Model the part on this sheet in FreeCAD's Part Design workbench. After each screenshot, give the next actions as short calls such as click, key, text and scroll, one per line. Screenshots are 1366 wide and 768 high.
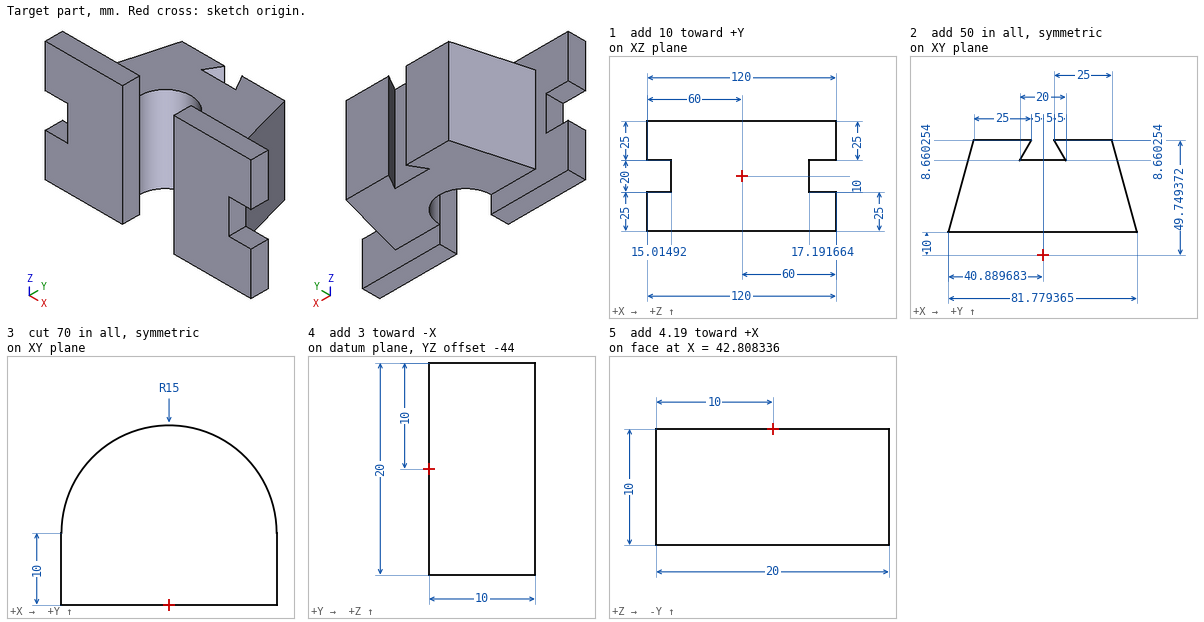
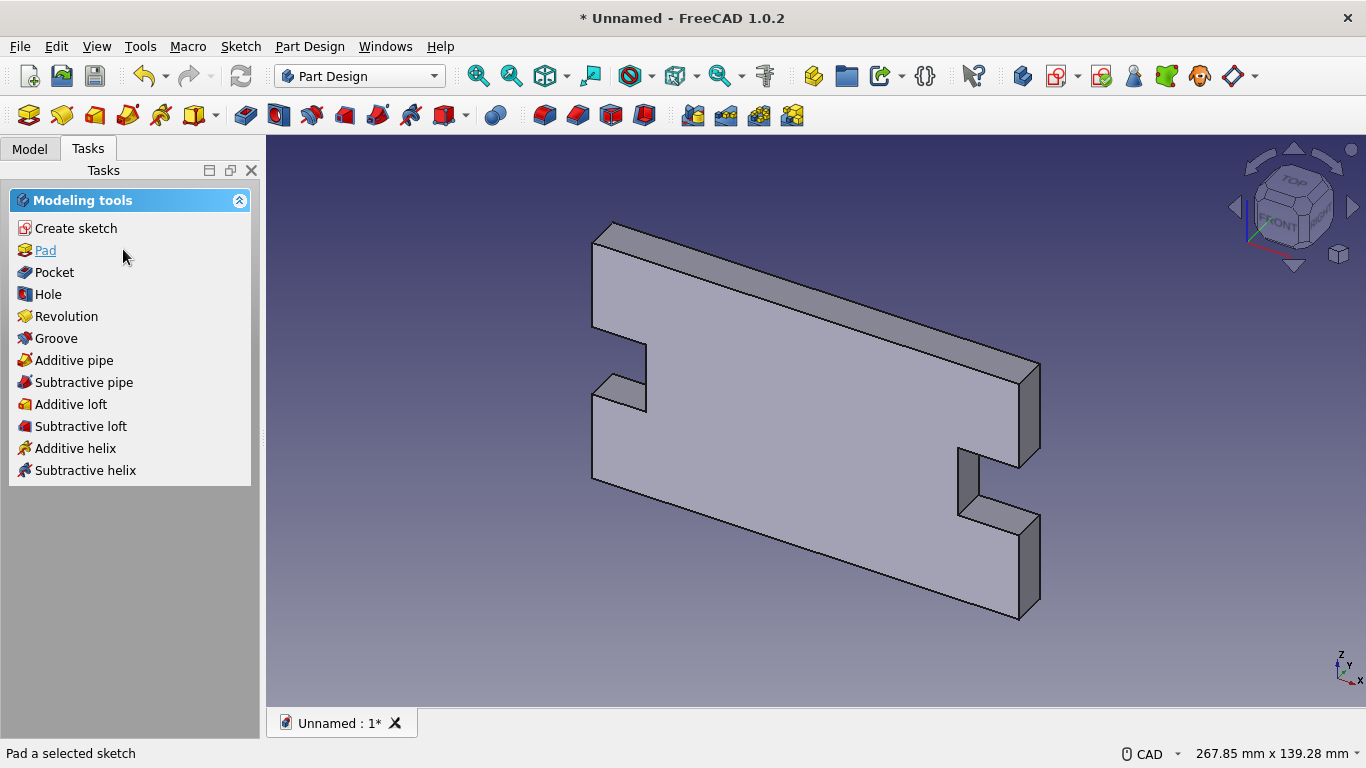
click(29, 116)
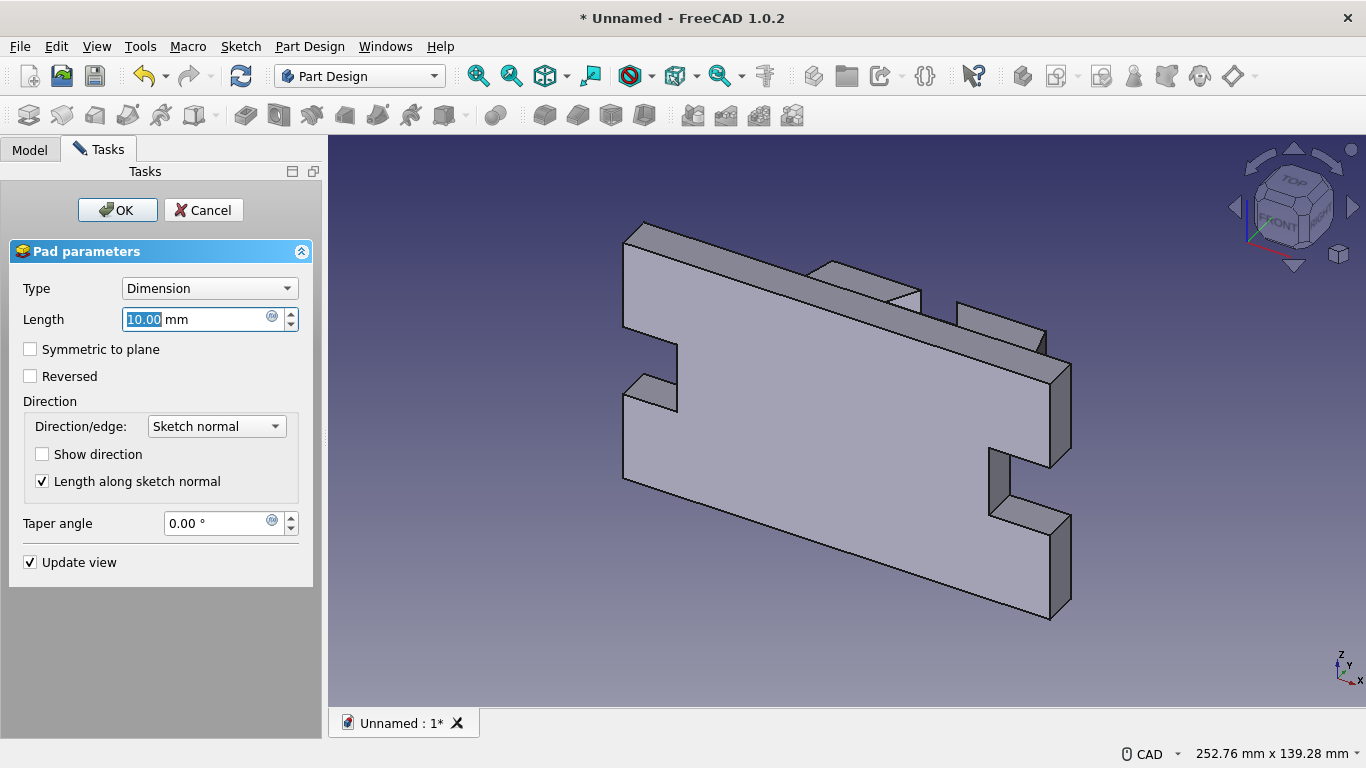
text(50)
key(Tab)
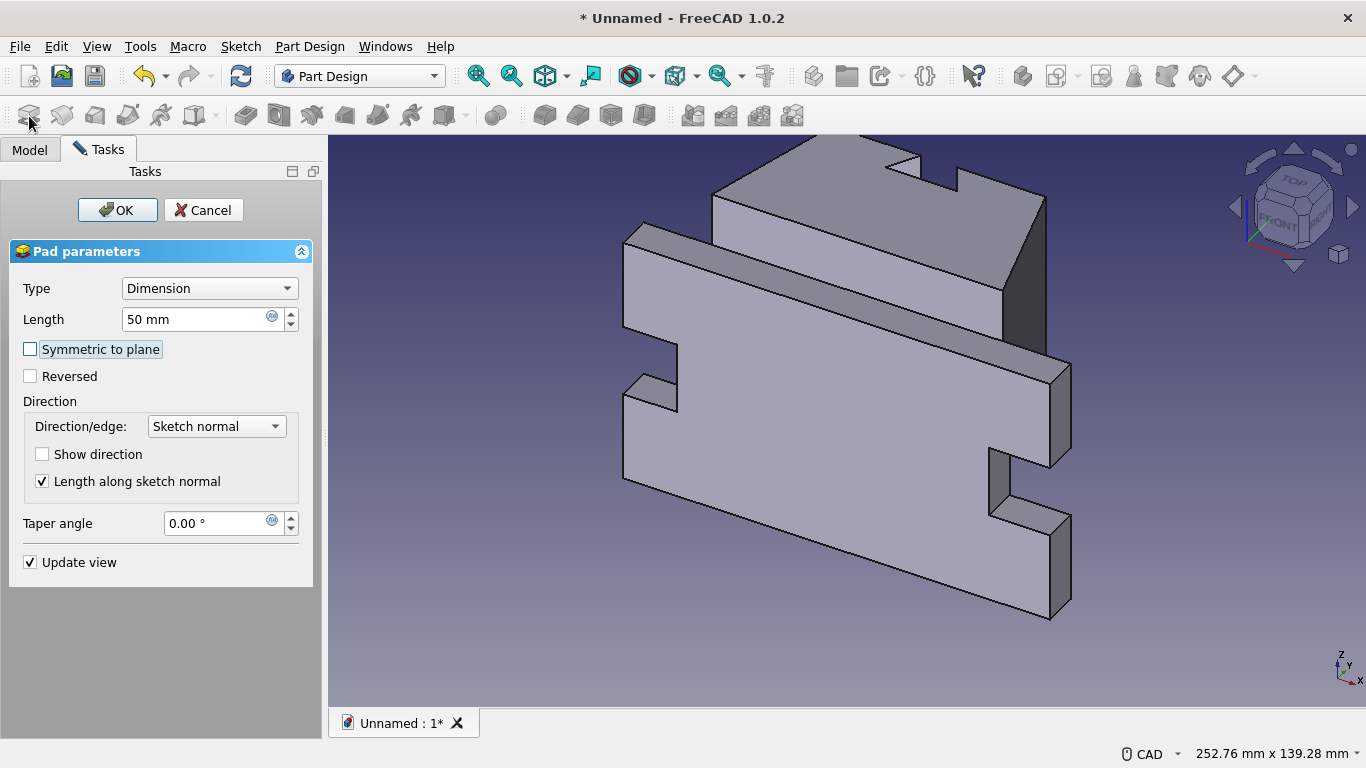
click(31, 349)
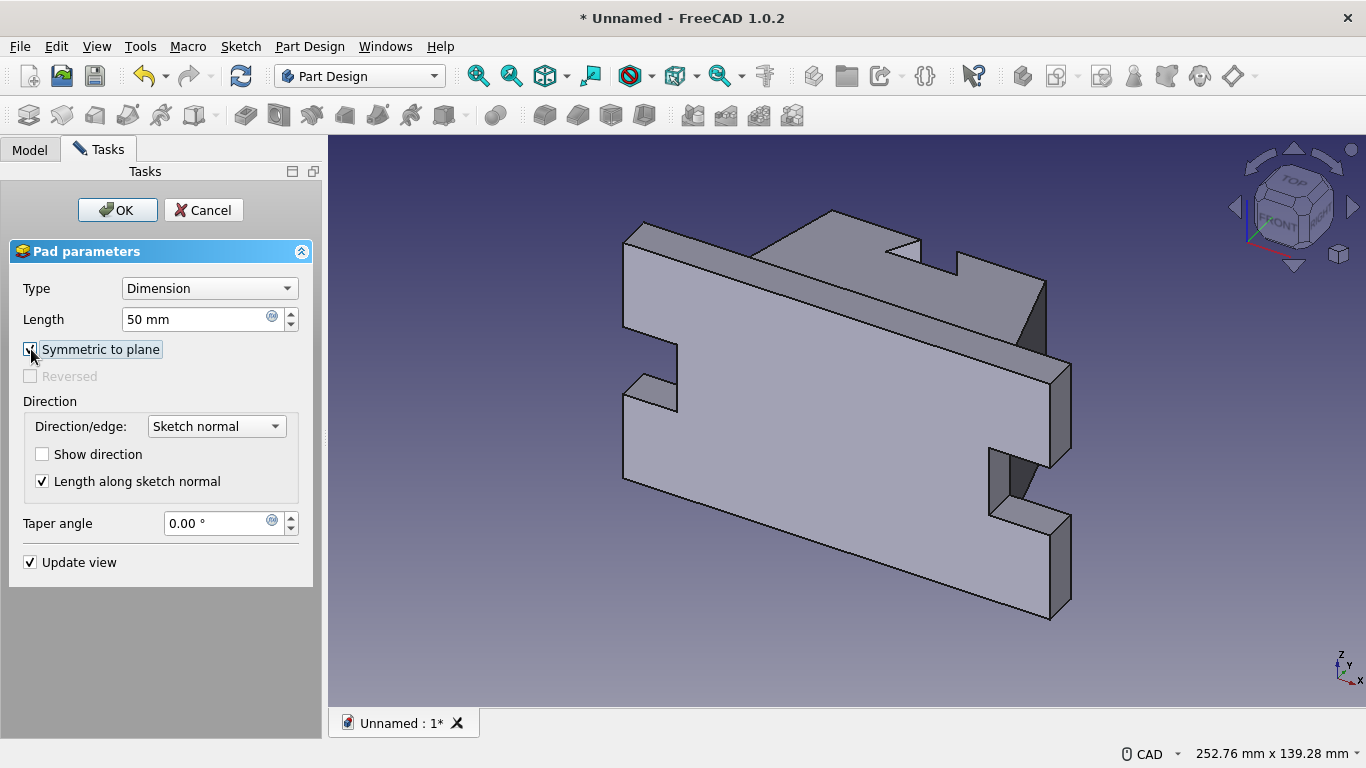
click(118, 210)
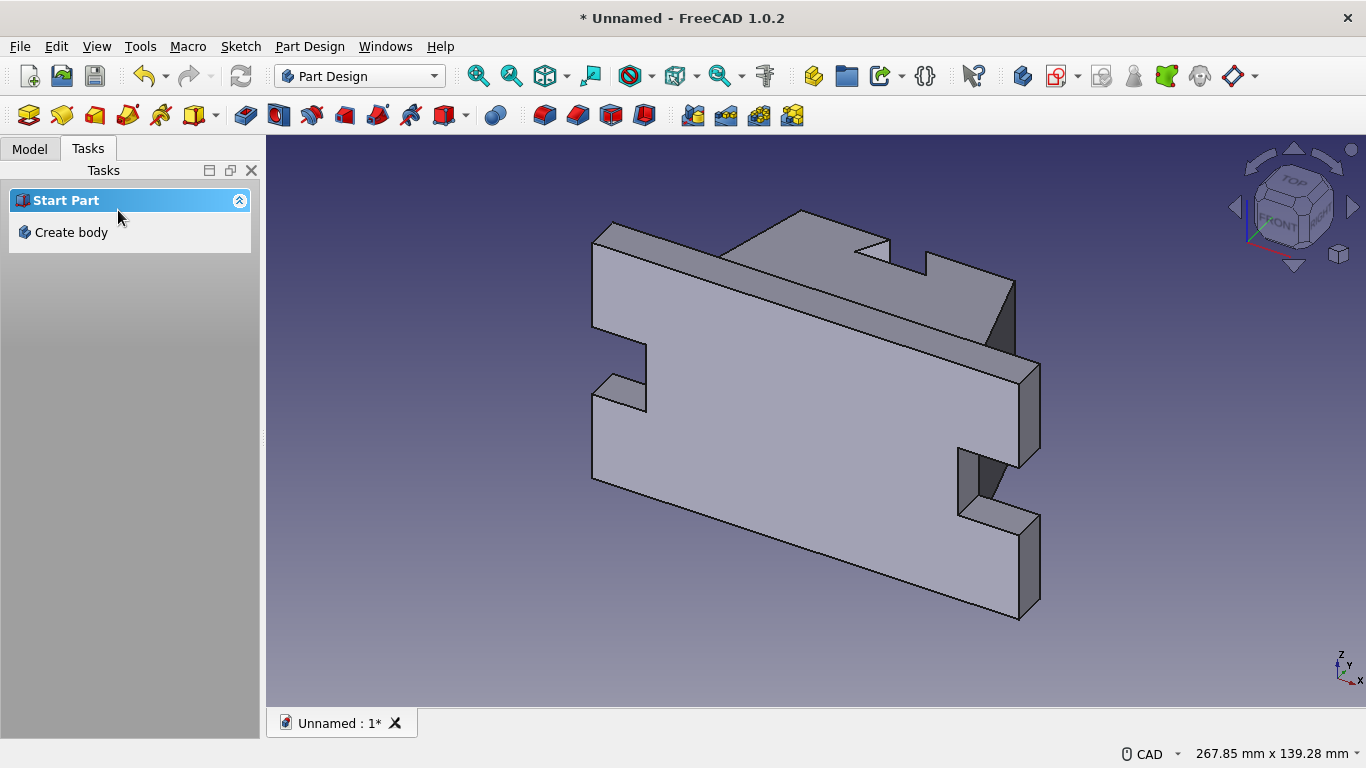
click(1056, 76)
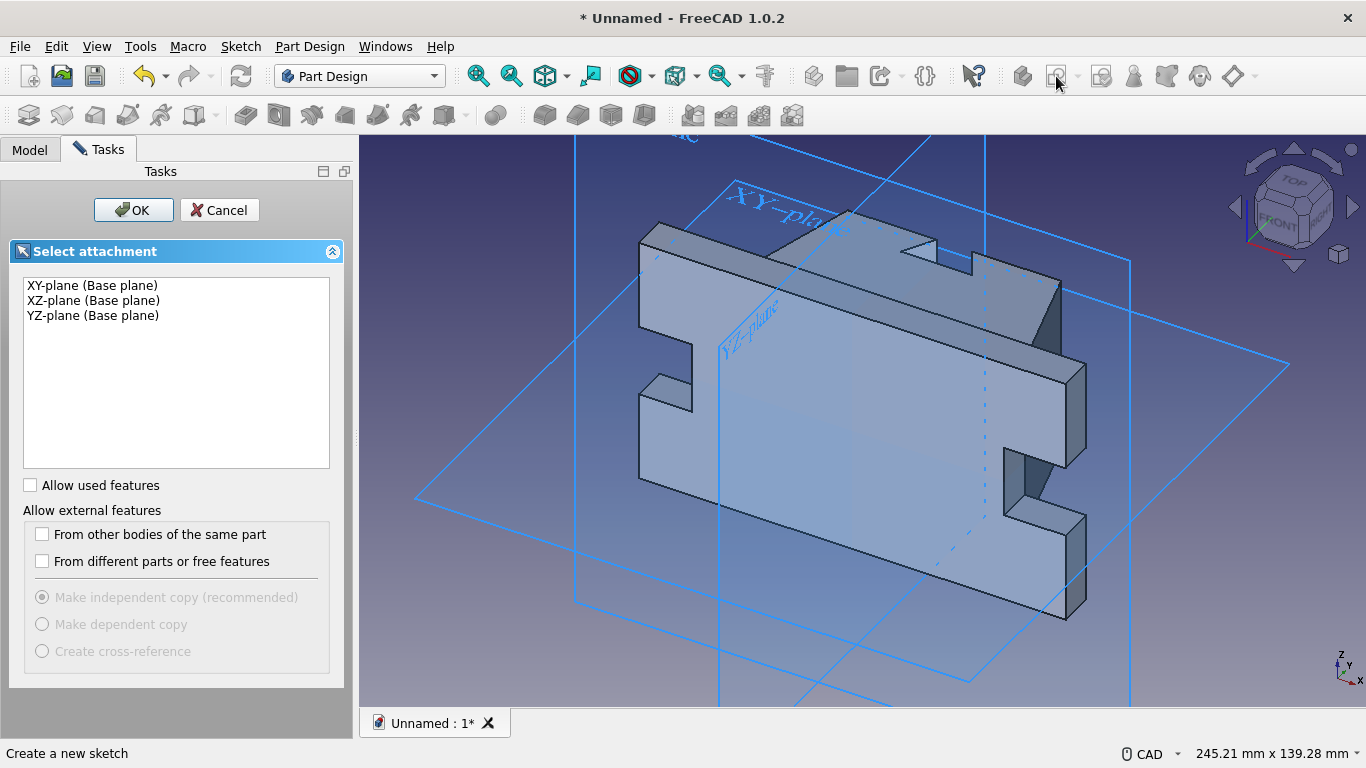
click(84, 286)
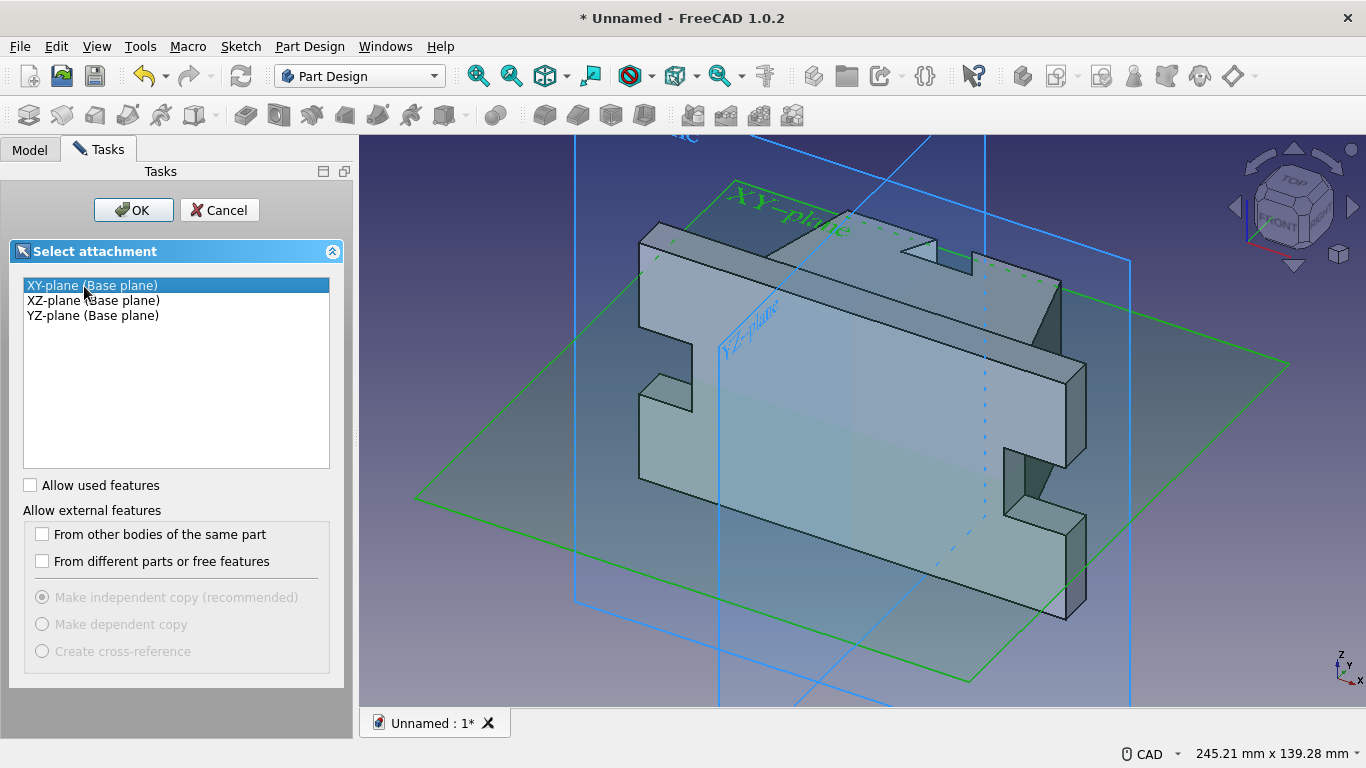
click(134, 210)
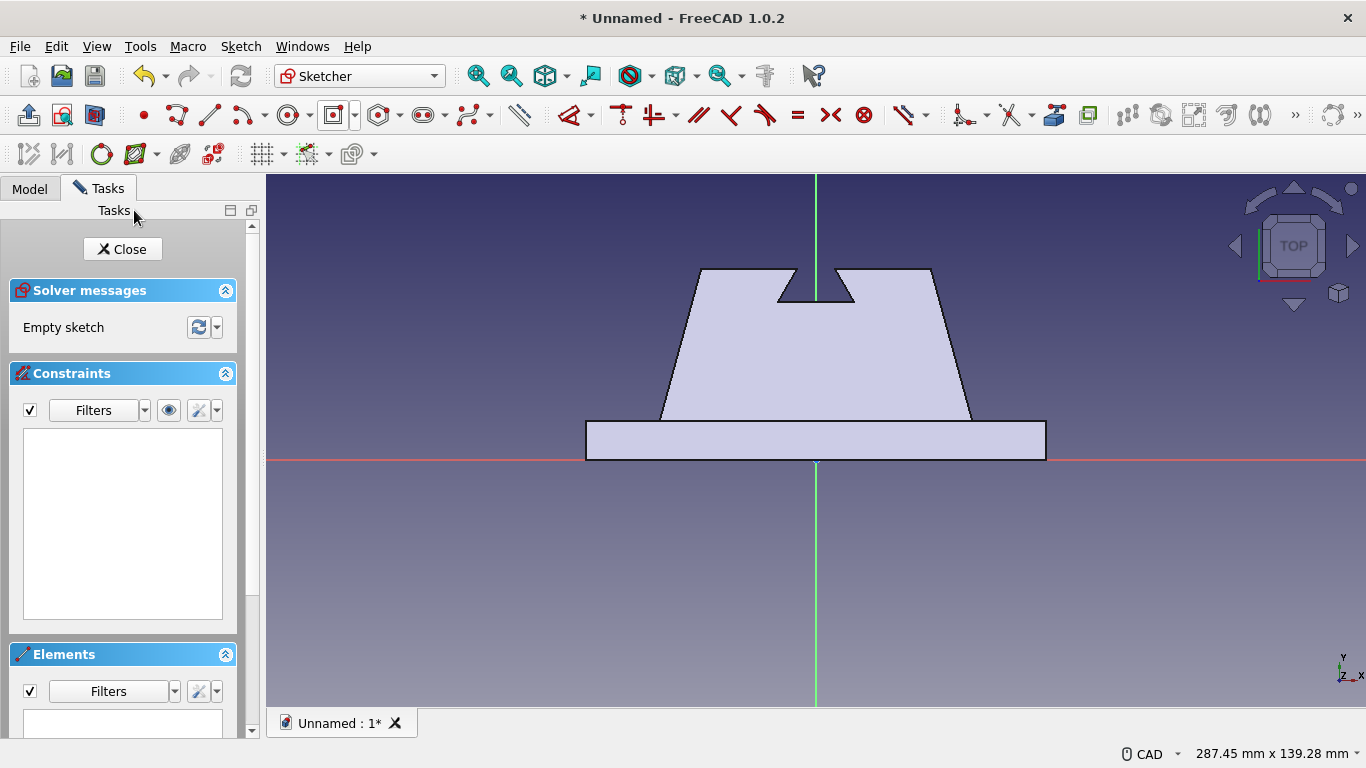
key(q)
key(s)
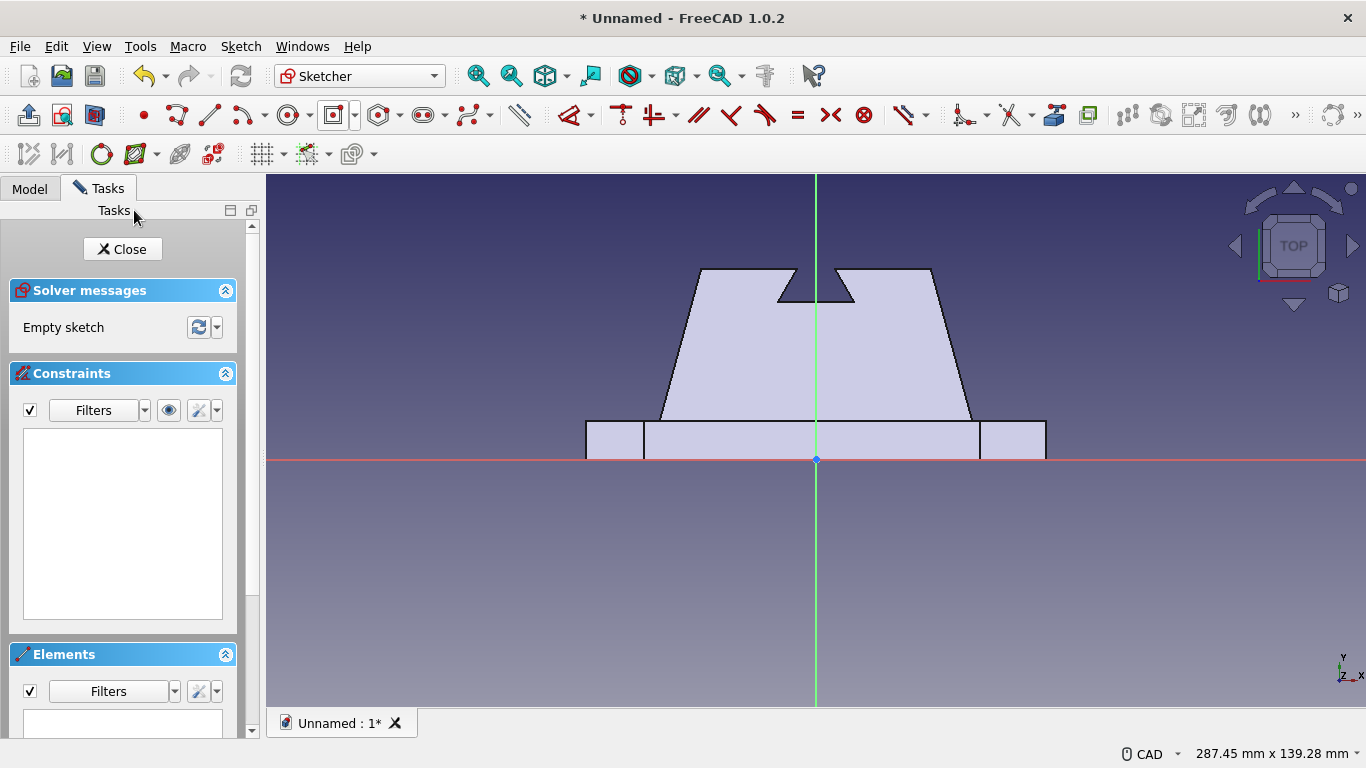
scroll(846, 399, up, 6)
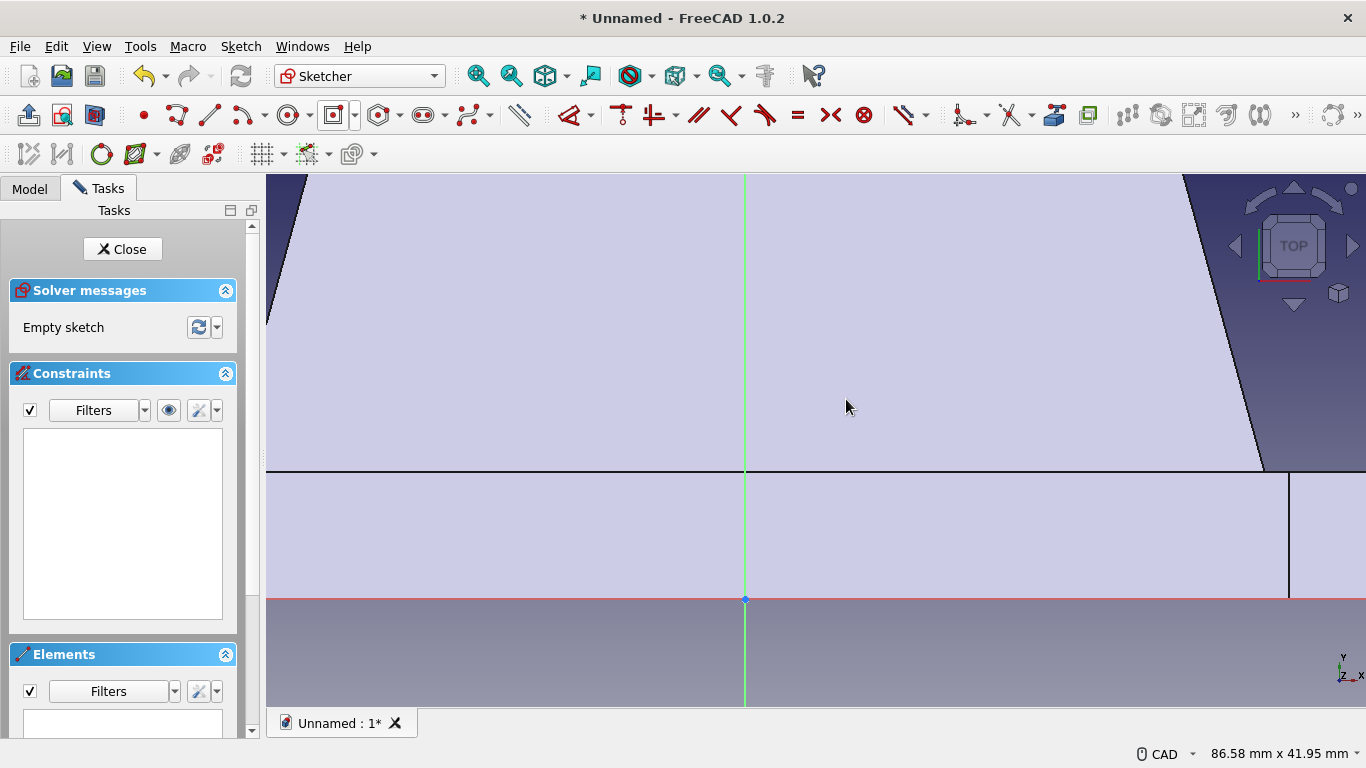
key(g)
key(m)